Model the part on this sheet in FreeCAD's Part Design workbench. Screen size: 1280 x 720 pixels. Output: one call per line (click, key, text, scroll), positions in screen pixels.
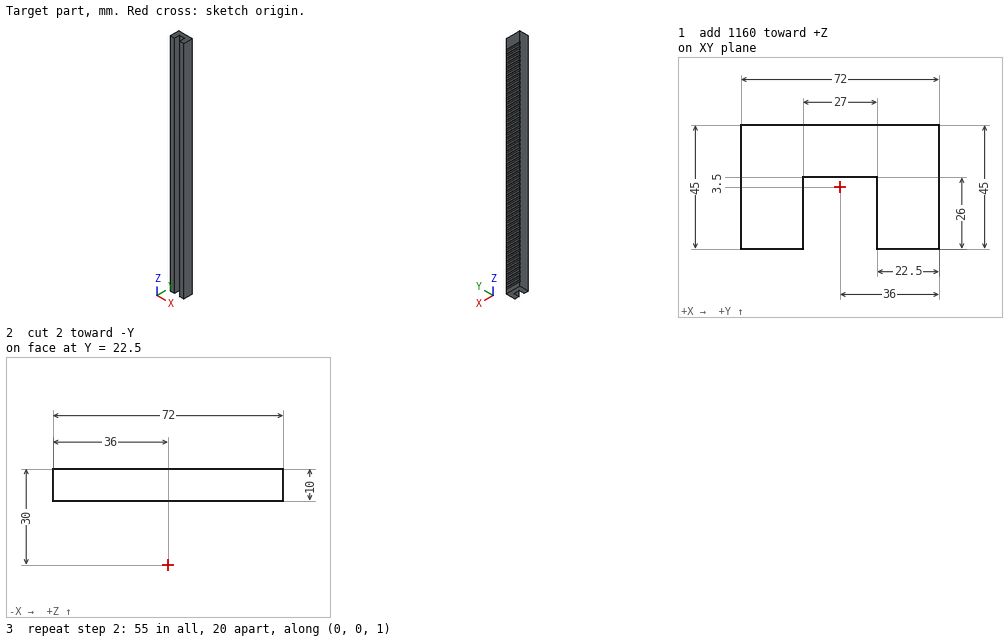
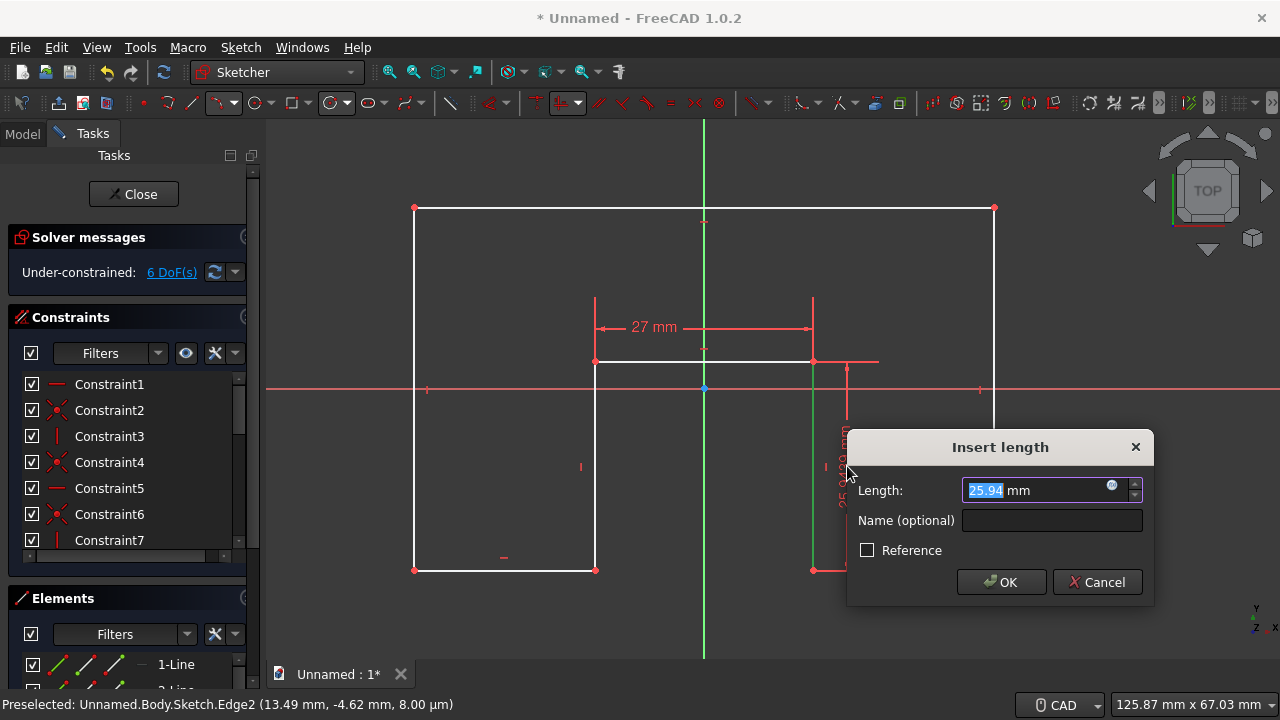
text(26)
key(Return)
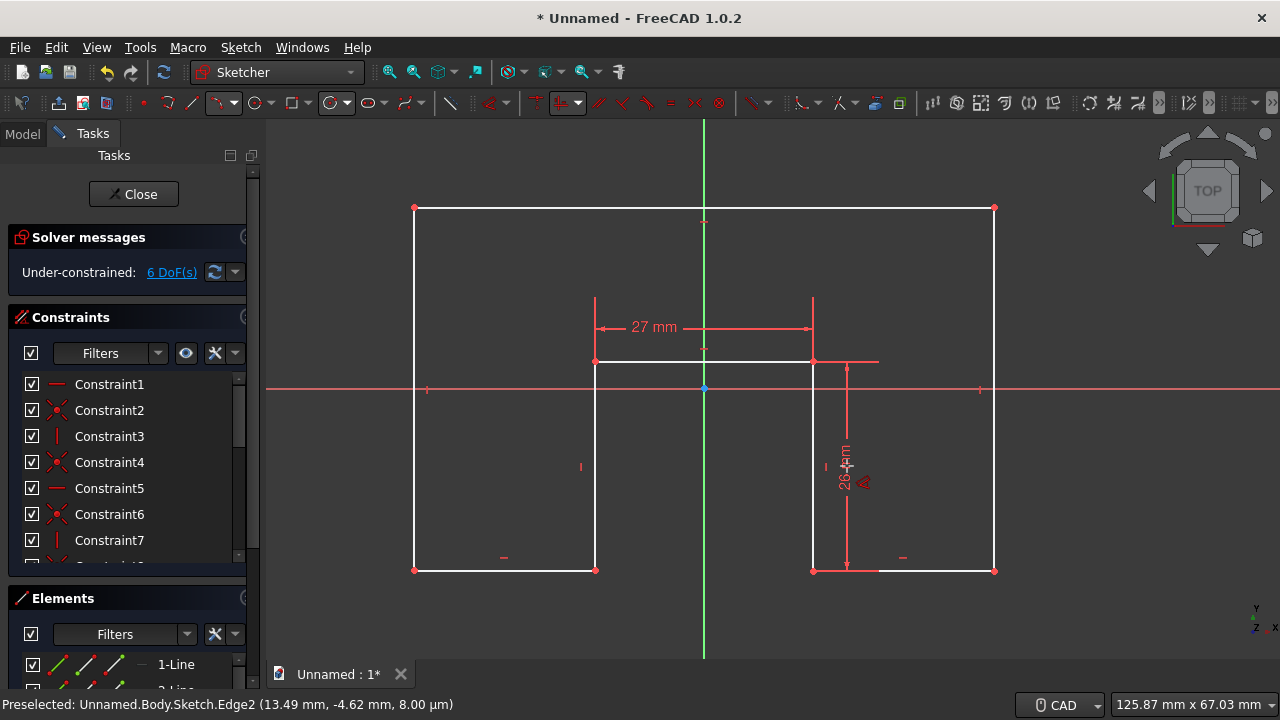
click(994, 462)
click(1028, 306)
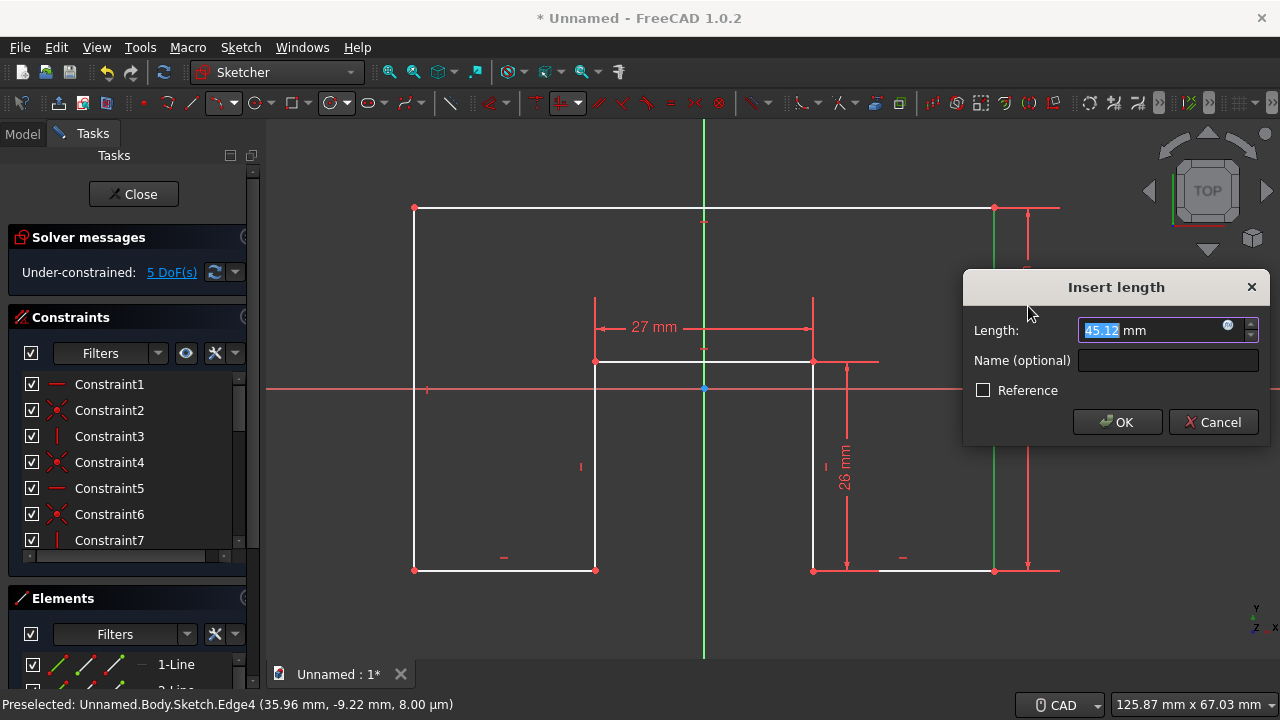
text(45)
key(Return)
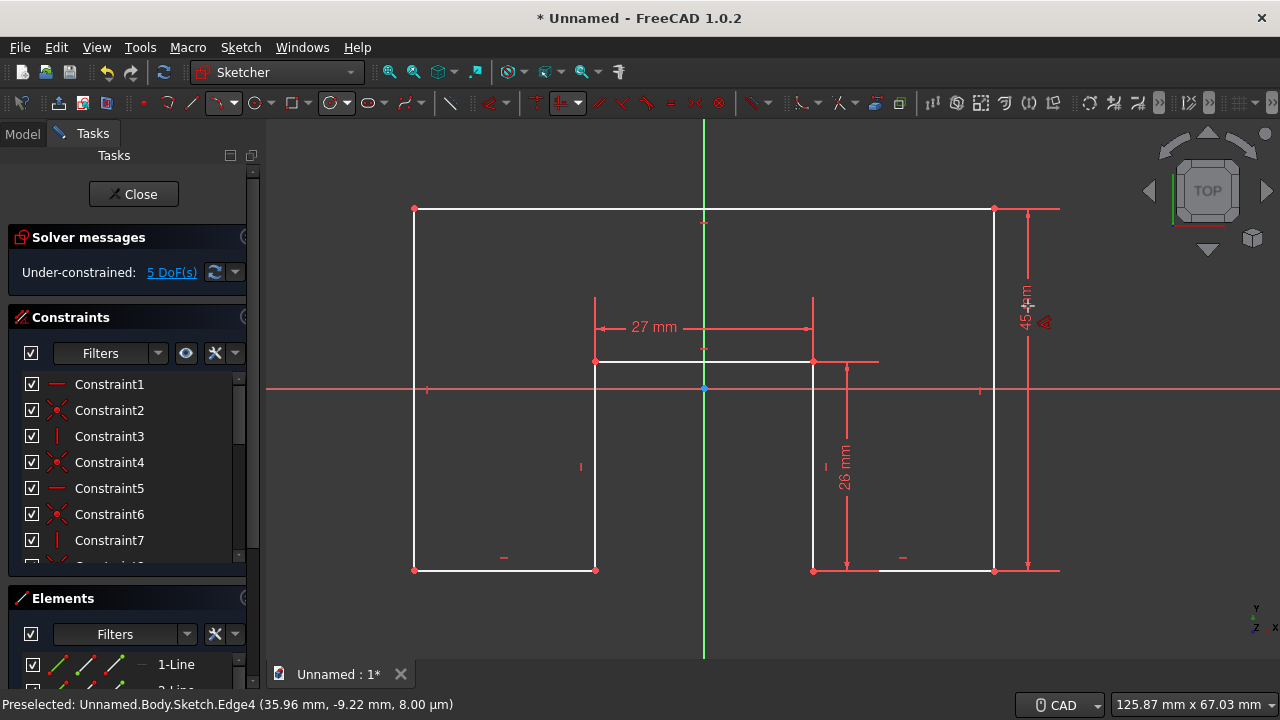
click(820, 209)
click(571, 175)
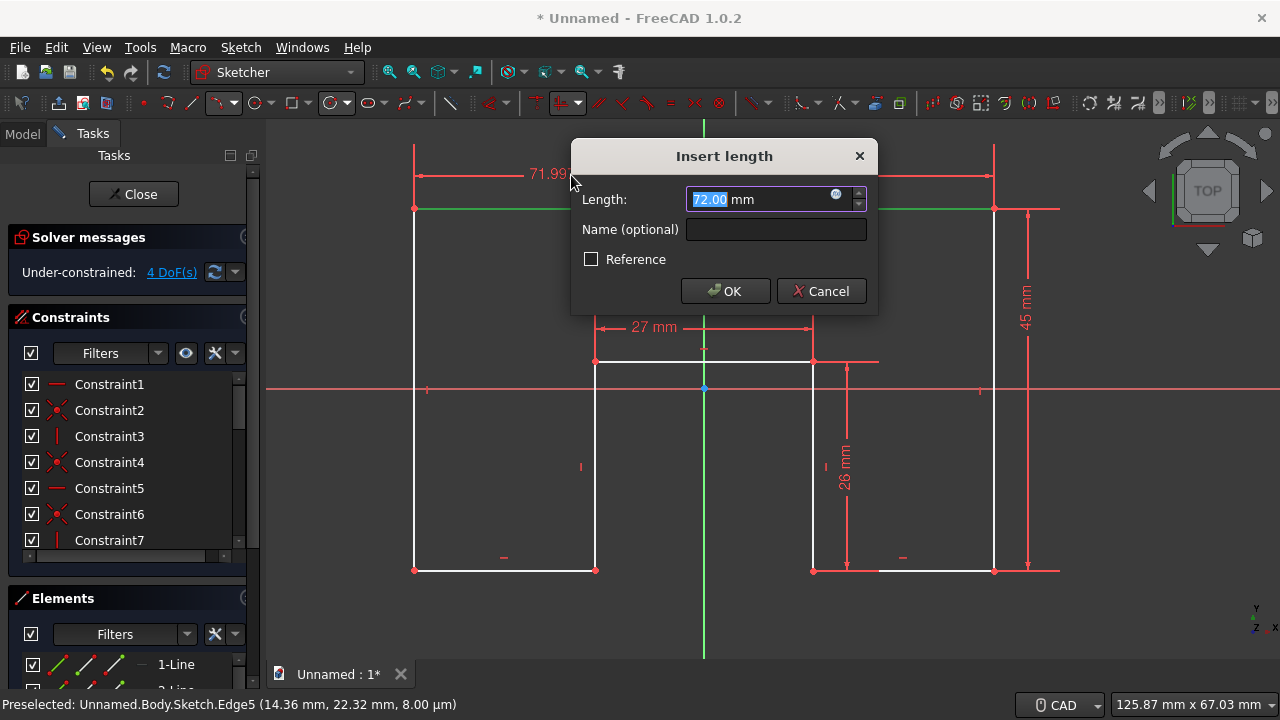
text(72)
key(Return)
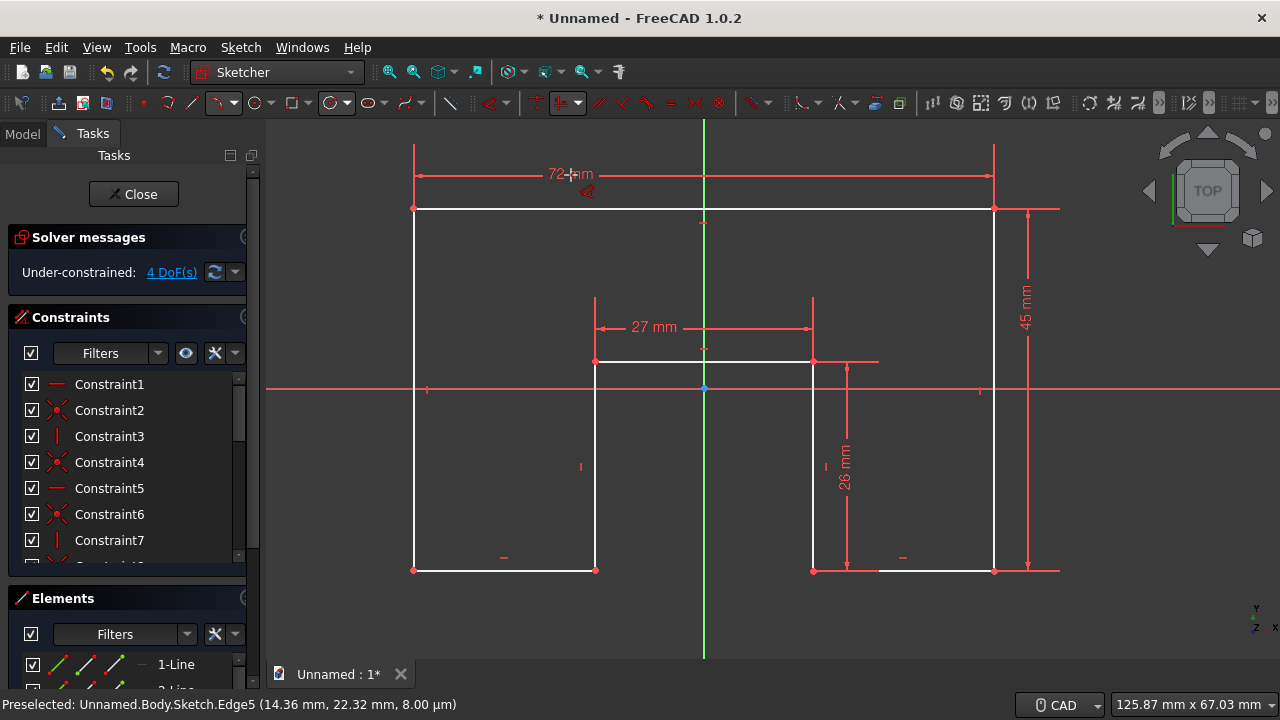
click(414, 318)
click(380, 307)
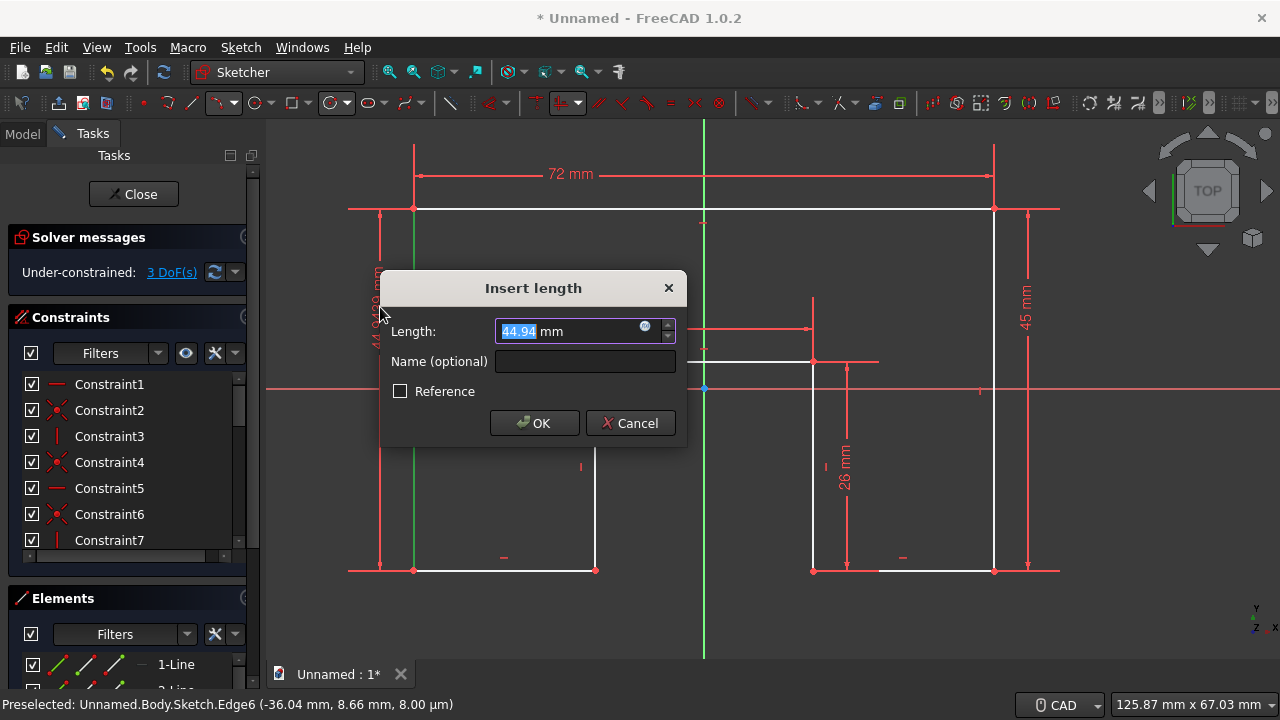
text(45)
key(Return)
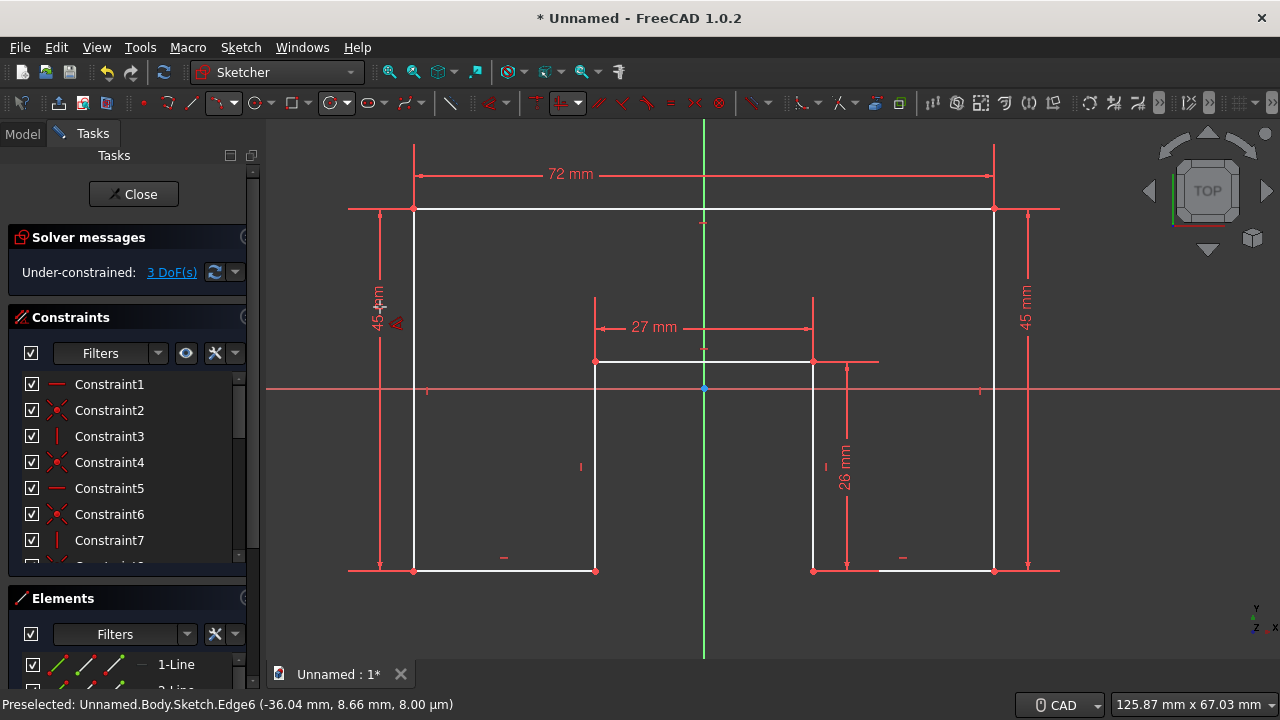
click(994, 571)
click(849, 605)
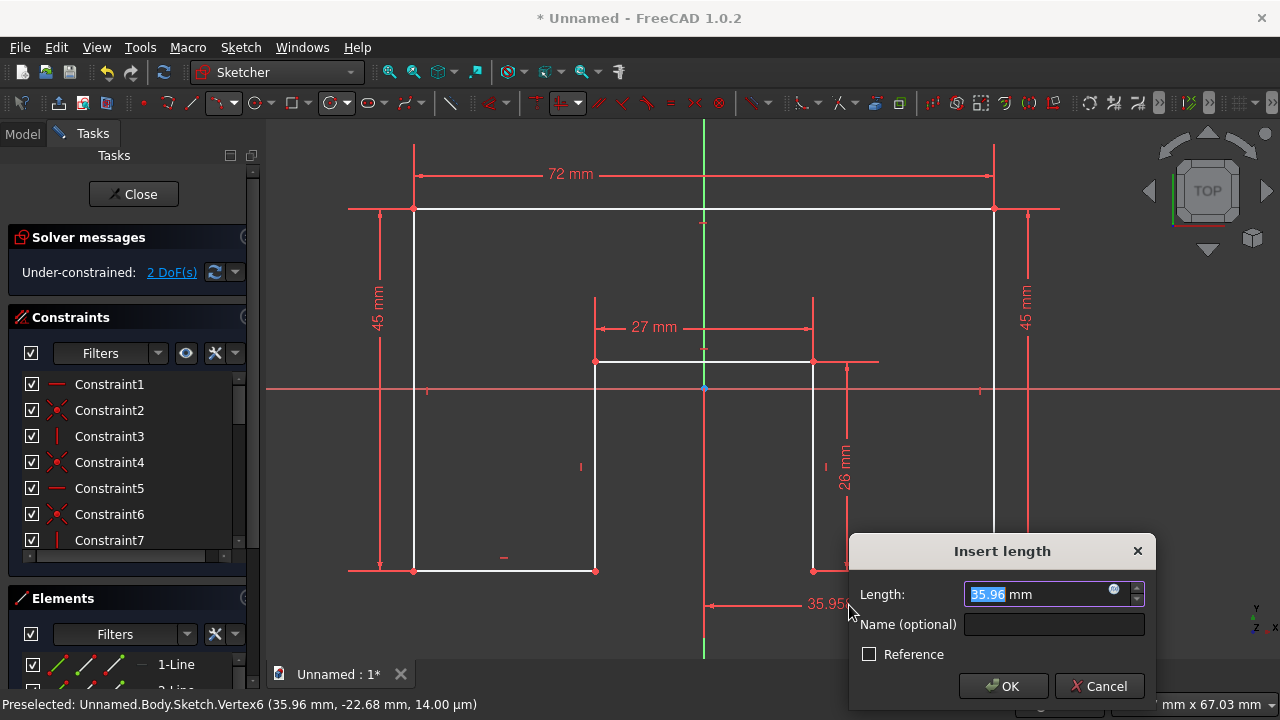
text(36)
key(Return)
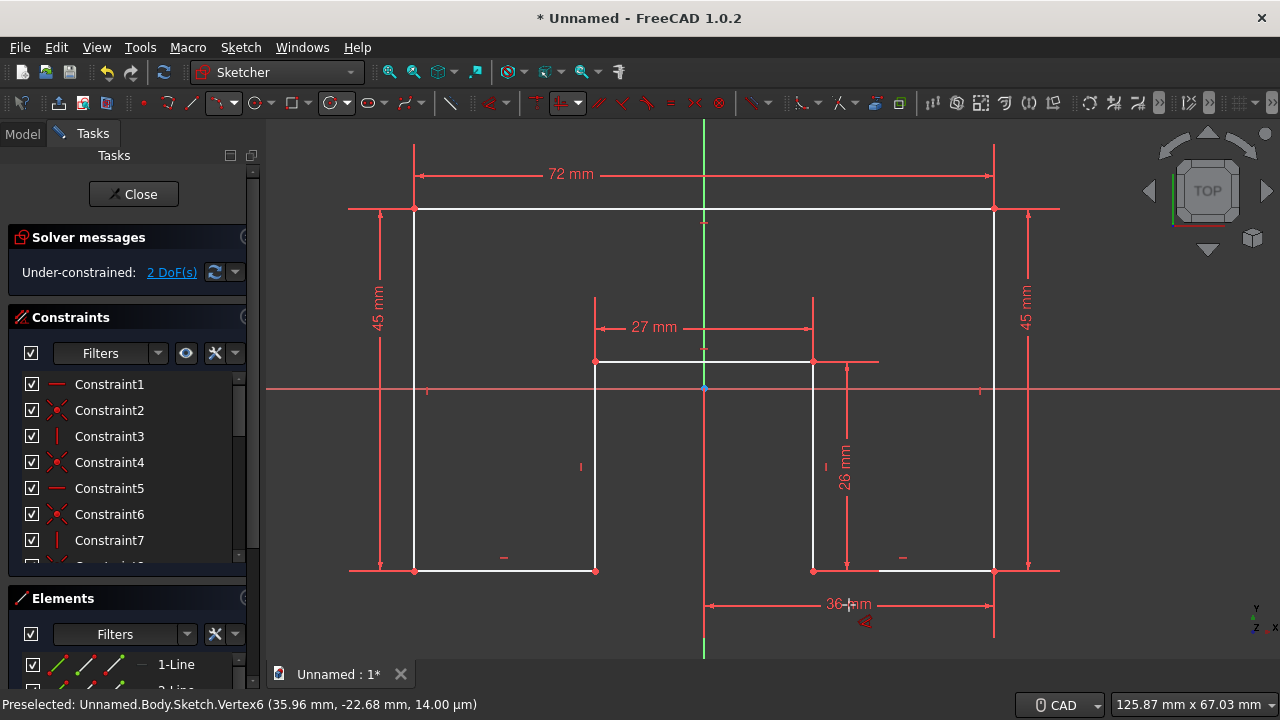
click(867, 571)
click(945, 605)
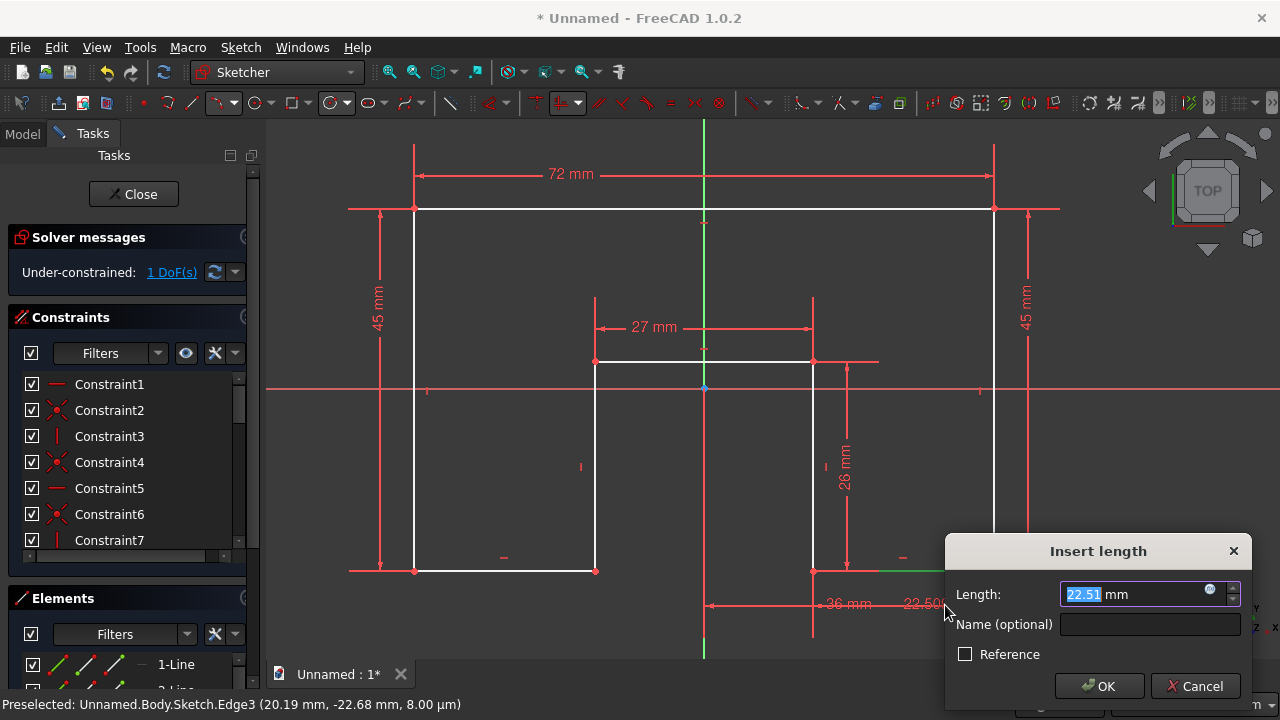
text(22.5)
key(Return)